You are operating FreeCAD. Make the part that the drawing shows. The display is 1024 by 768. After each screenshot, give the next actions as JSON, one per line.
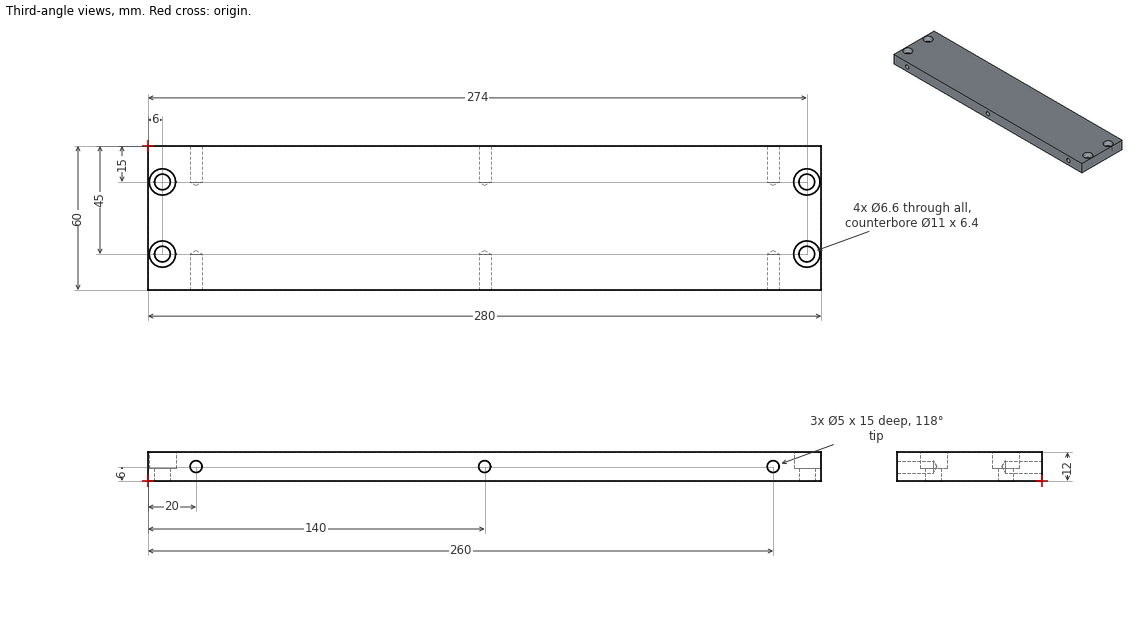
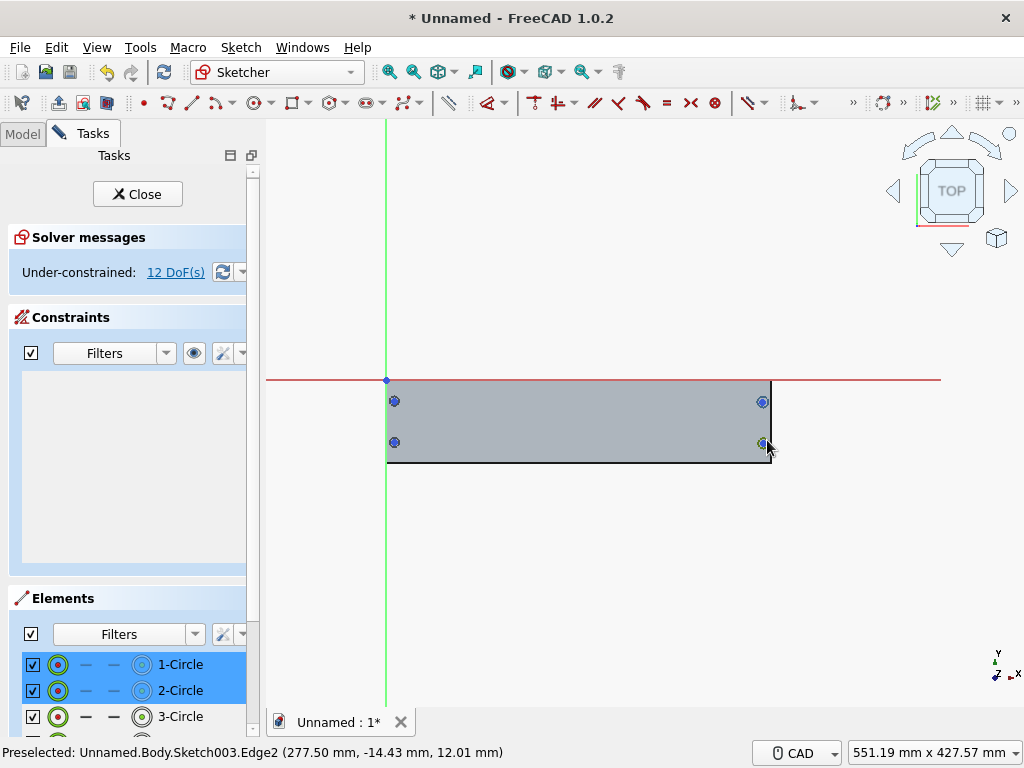
{"action": "scroll", "coordinate": [398, 439], "scroll_direction": "up", "scroll_amount": 6}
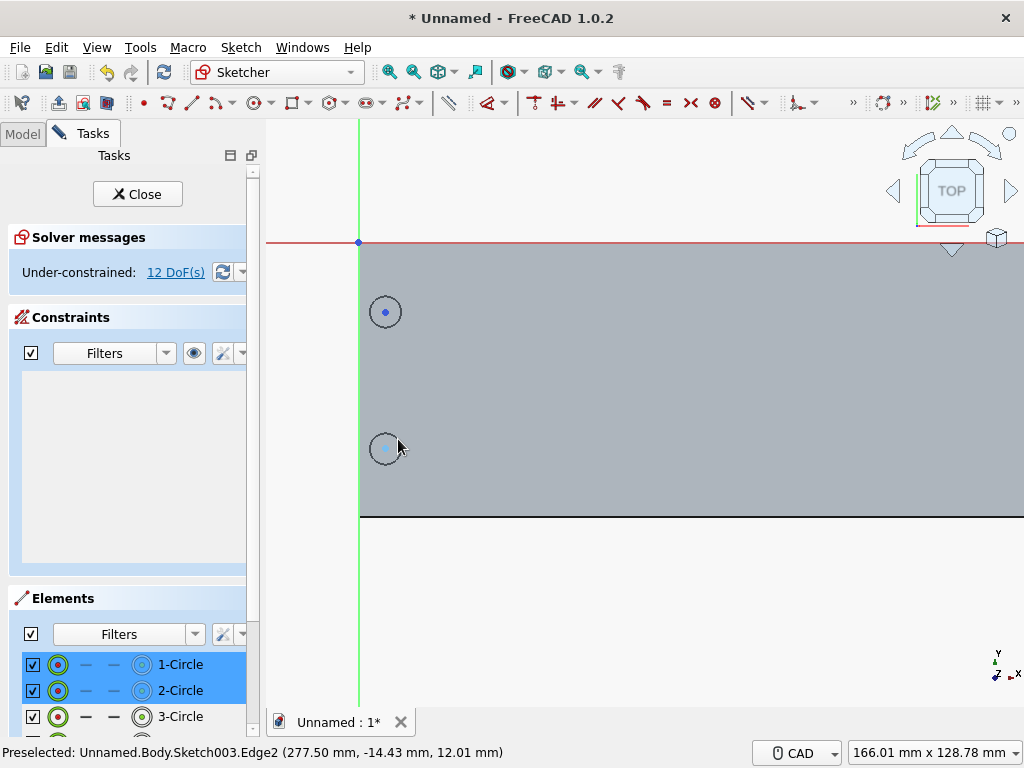
{"action": "left_click", "coordinate": [396, 438]}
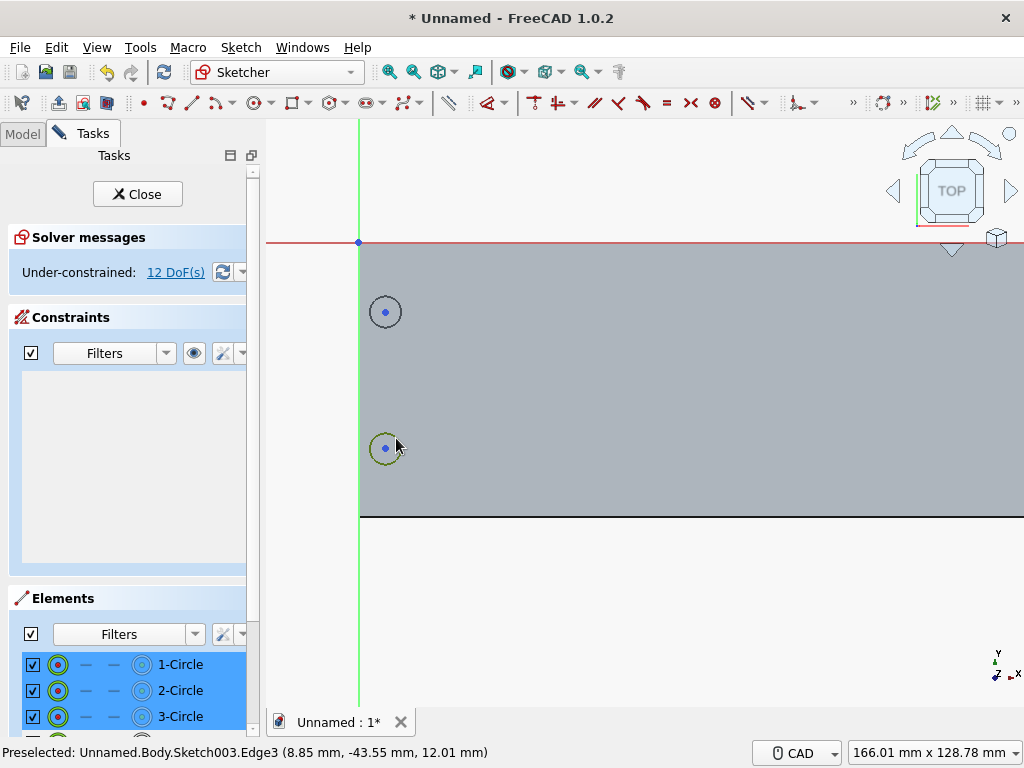
{"action": "left_click", "coordinate": [397, 301]}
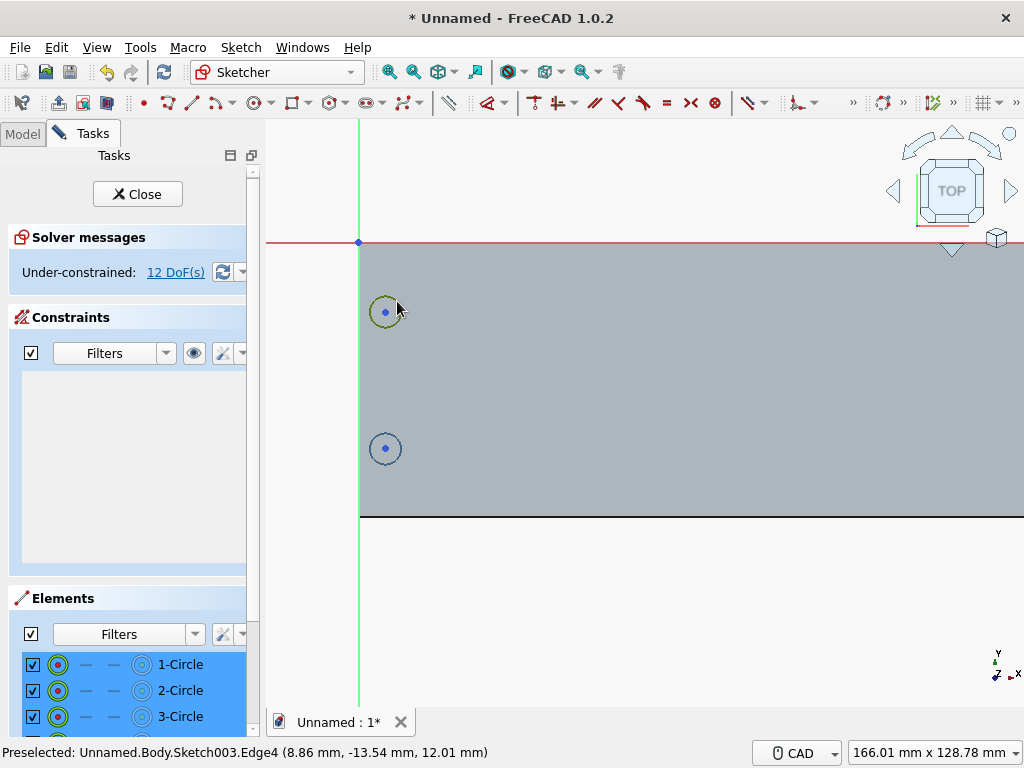
{"action": "left_click", "coordinate": [668, 104]}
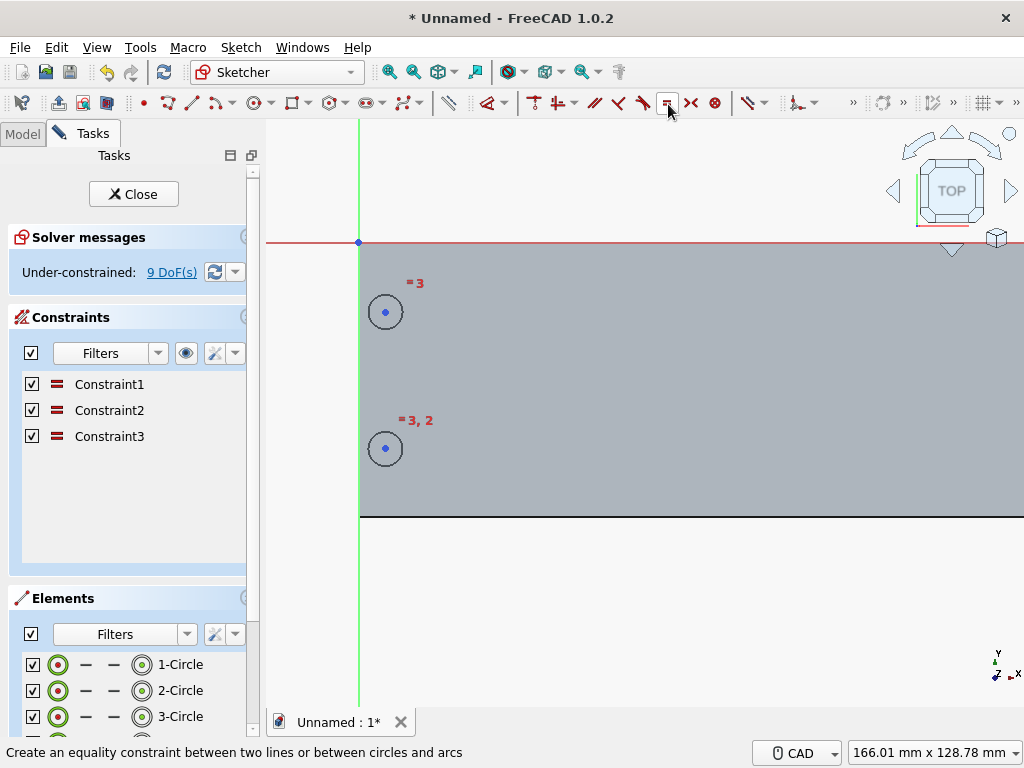
{"action": "left_click", "coordinate": [488, 104]}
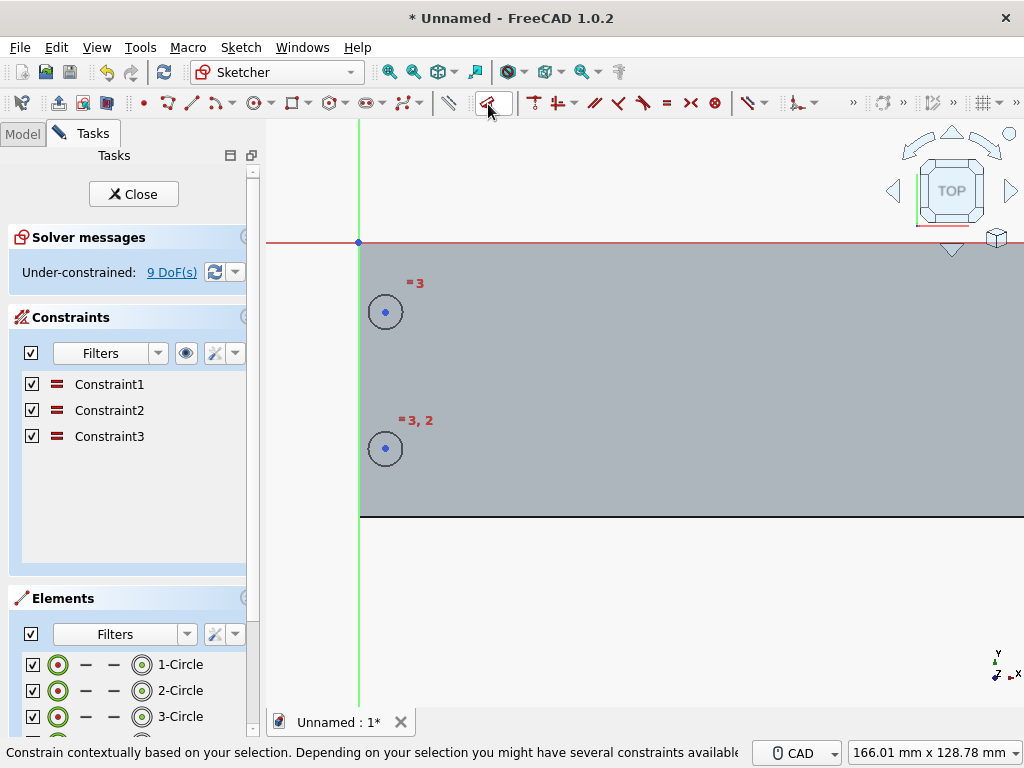
{"action": "scroll", "coordinate": [398, 439], "scroll_direction": "down", "scroll_amount": 6}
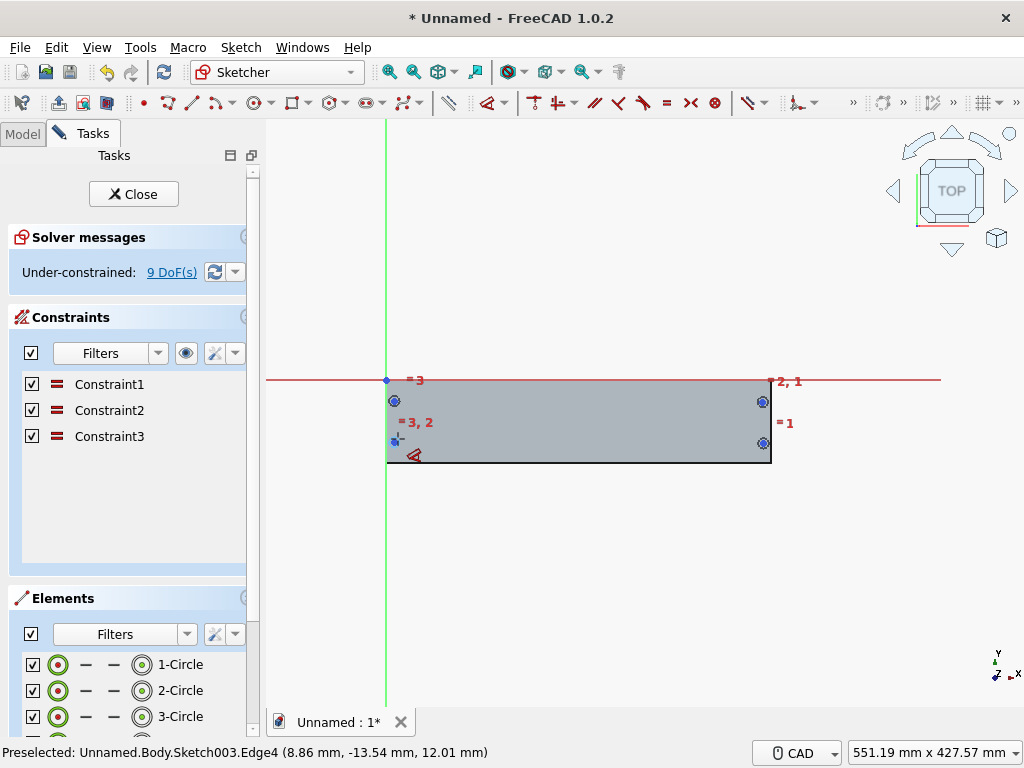
{"action": "scroll", "coordinate": [767, 440], "scroll_direction": "up", "scroll_amount": 8}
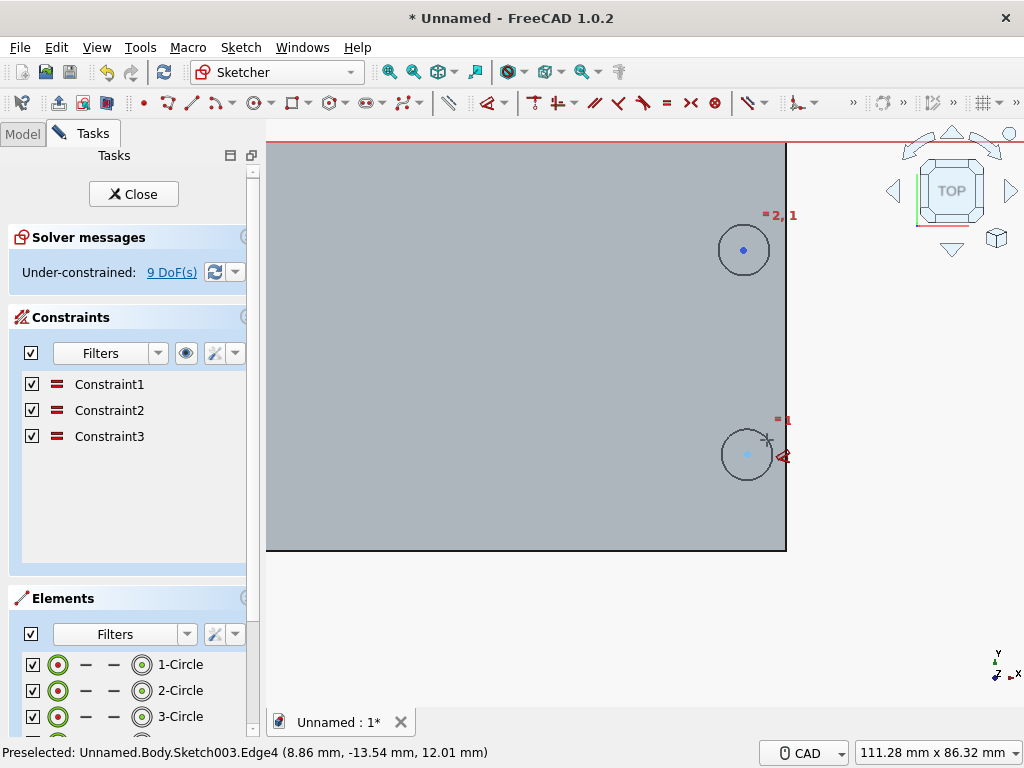
{"action": "left_click", "coordinate": [765, 437]}
{"action": "left_click", "coordinate": [788, 415]}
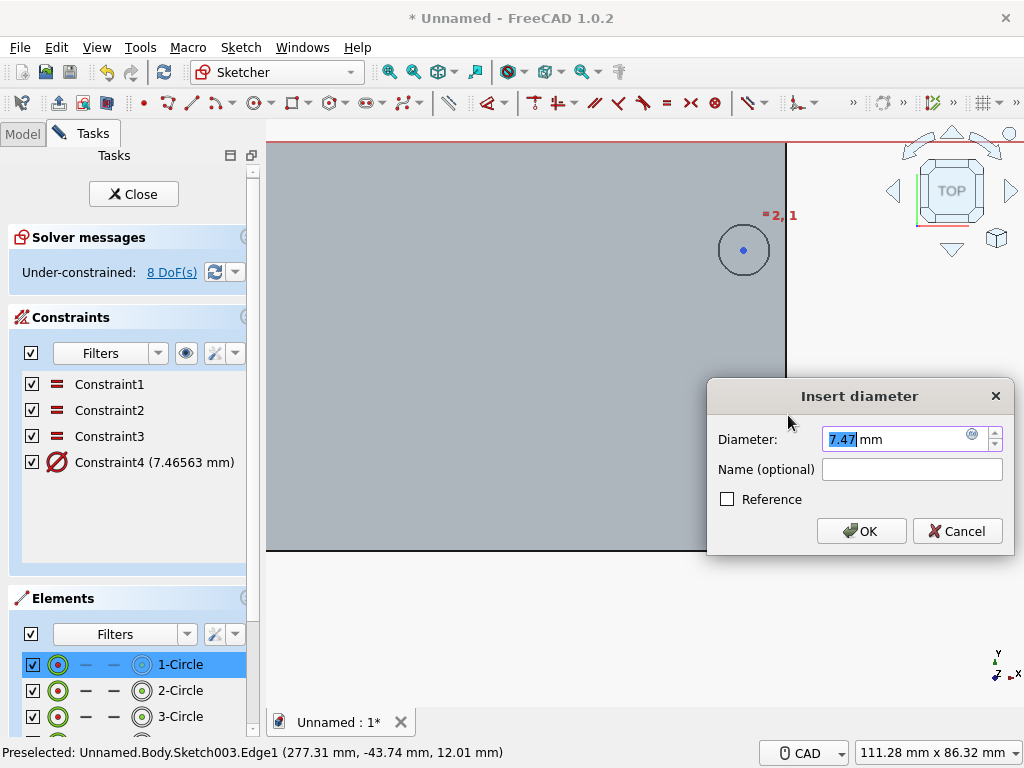
{"action": "type", "text": "6.6"}
{"action": "key", "text": "Return"}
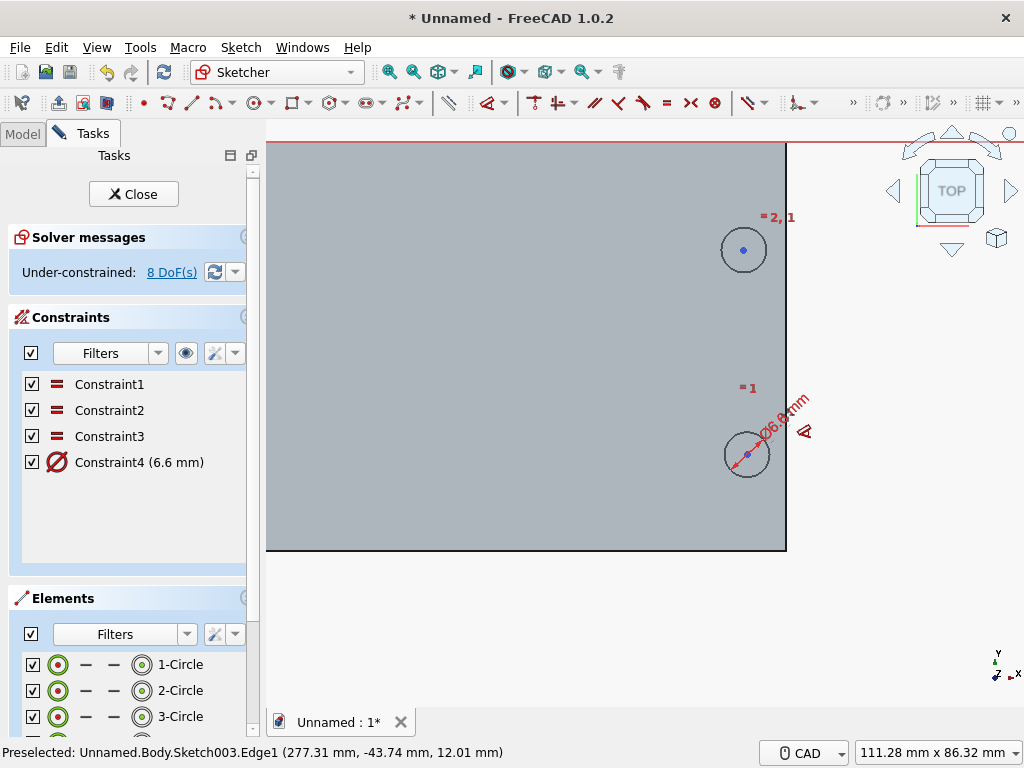
{"action": "scroll", "coordinate": [767, 440], "scroll_direction": "down", "scroll_amount": 8}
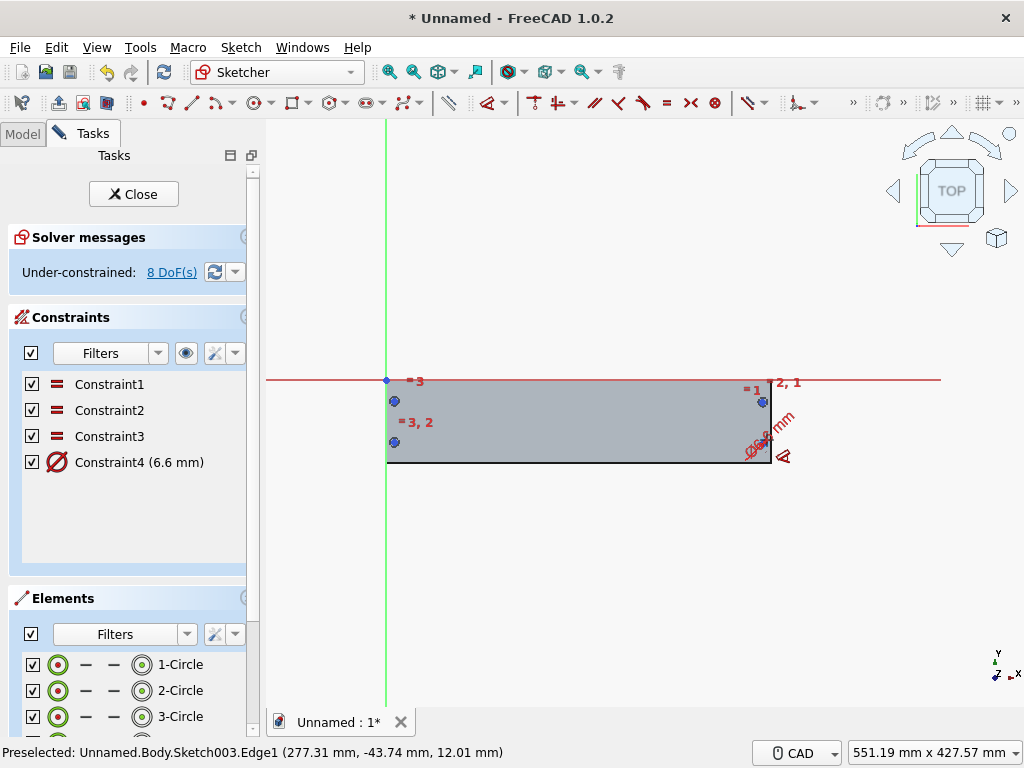
{"action": "scroll", "coordinate": [394, 442], "scroll_direction": "up", "scroll_amount": 8}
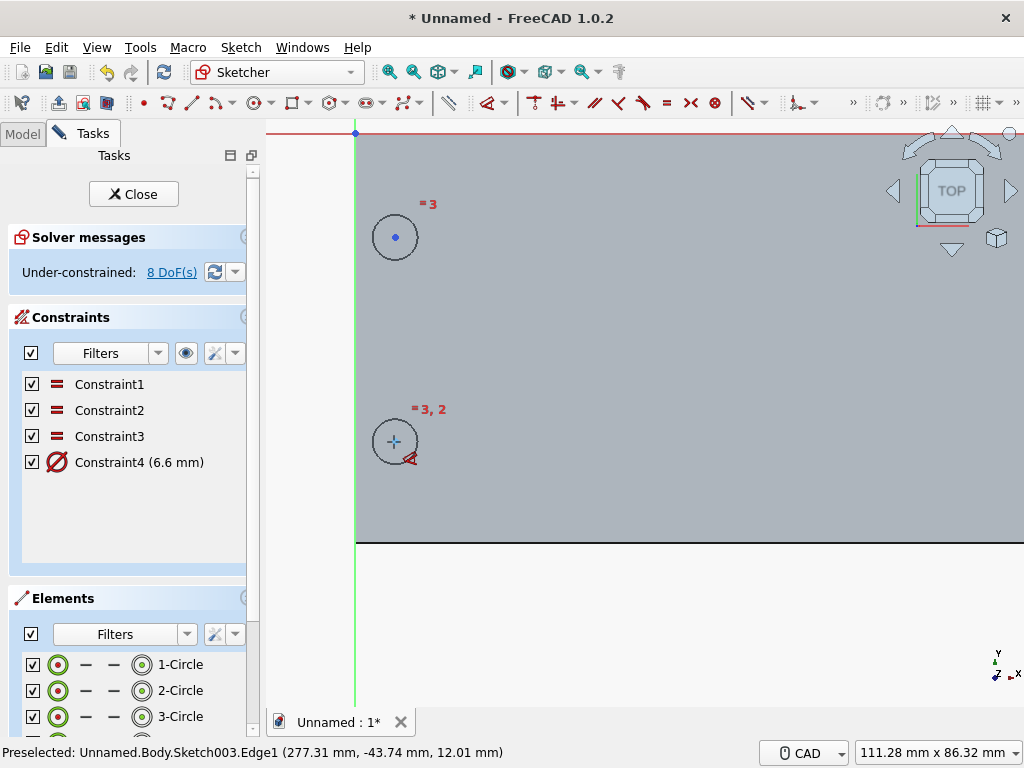
{"action": "left_click", "coordinate": [395, 442]}
{"action": "left_click", "coordinate": [375, 476]}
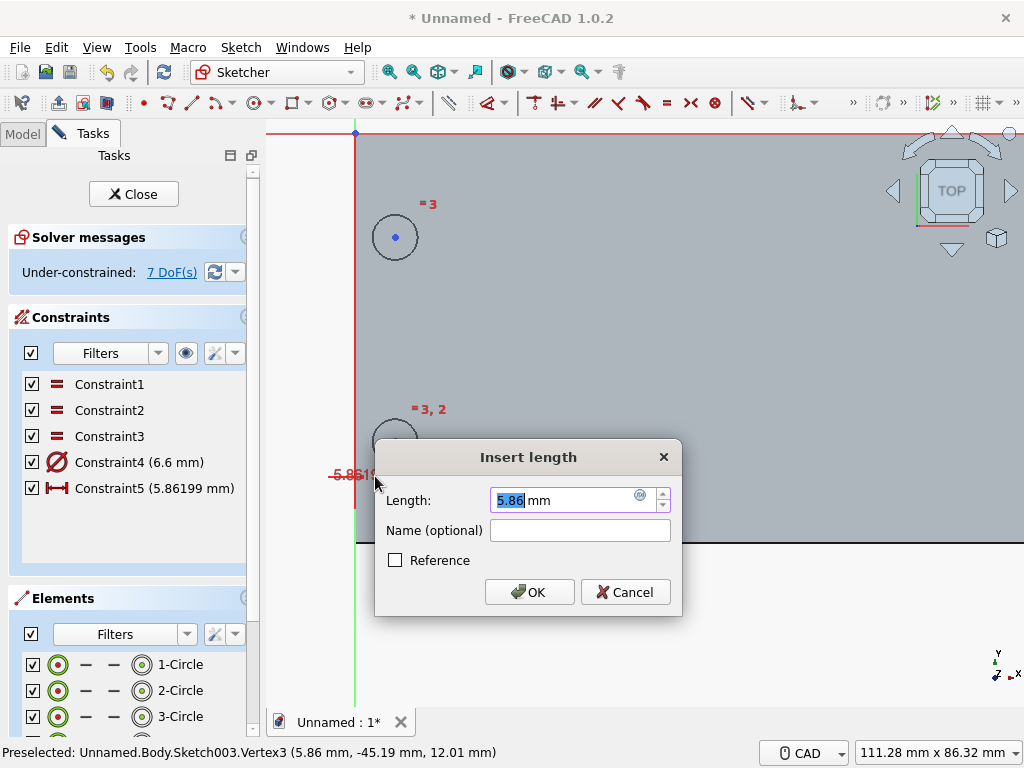
{"action": "type", "text": "6"}
{"action": "key", "text": "Return"}